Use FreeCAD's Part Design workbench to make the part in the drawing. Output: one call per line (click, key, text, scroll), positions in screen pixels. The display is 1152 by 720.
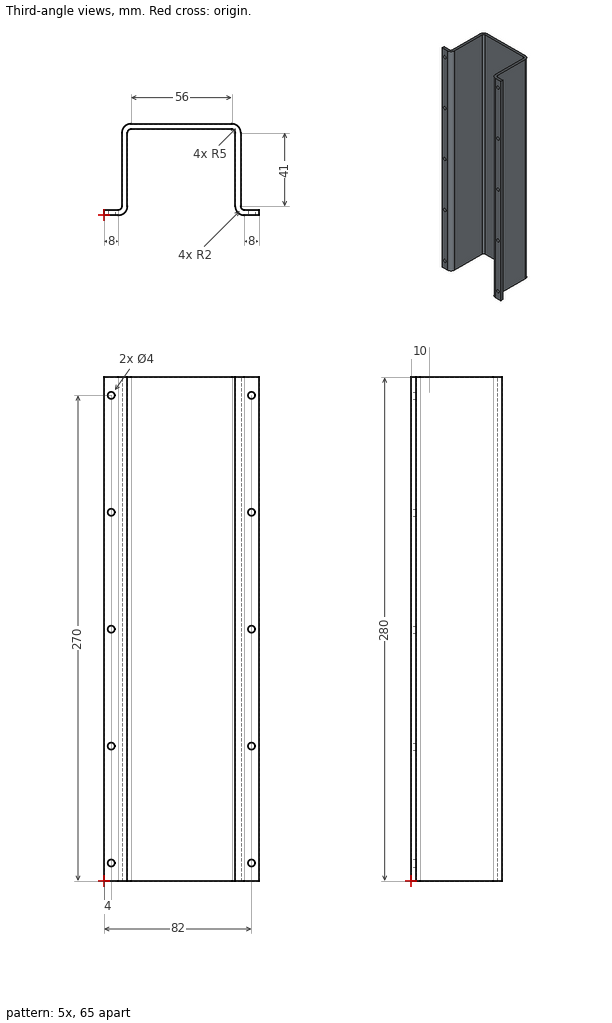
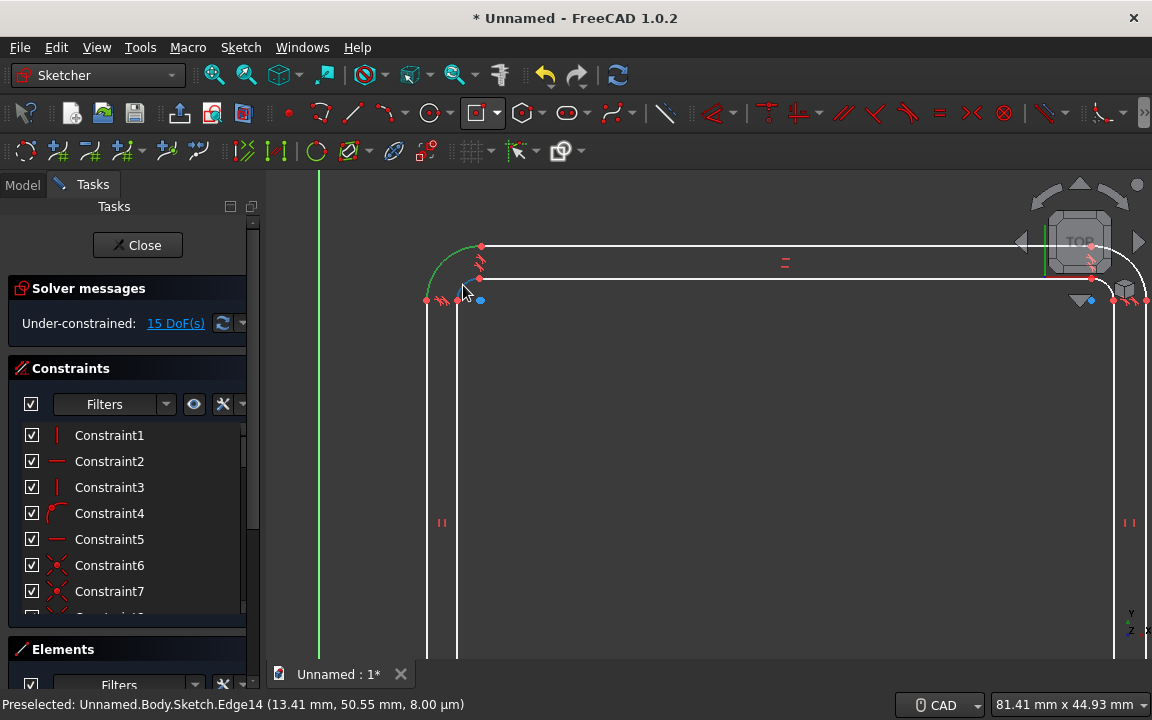
click(464, 285)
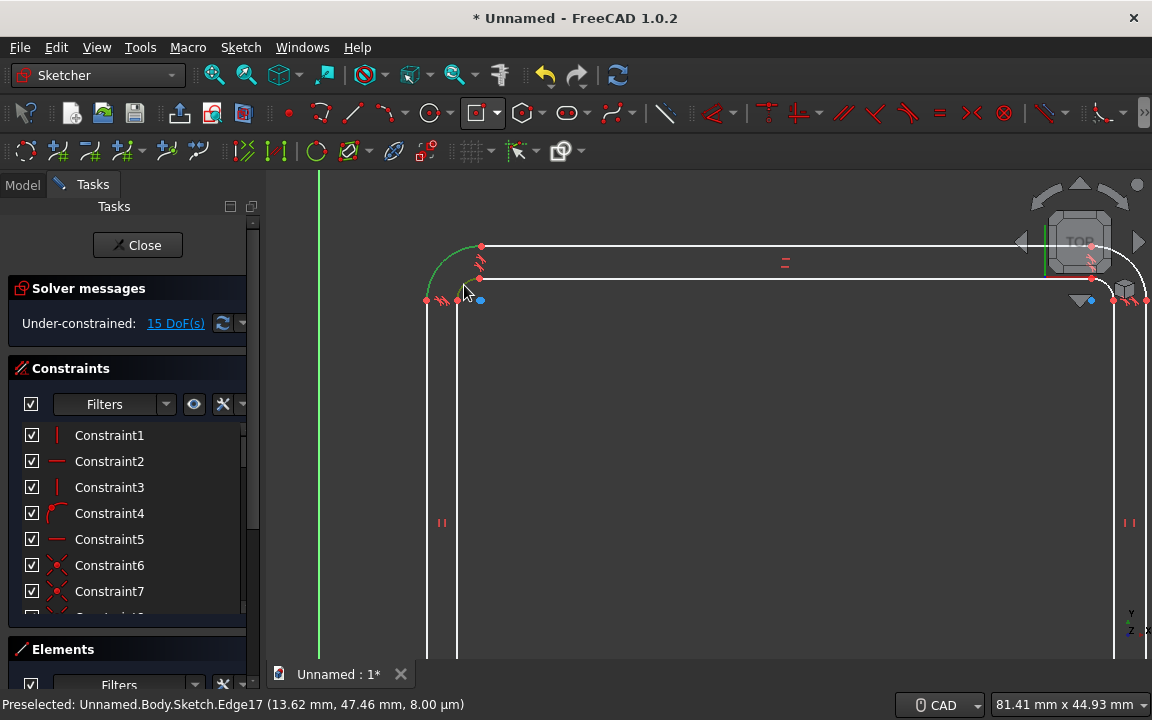
key(c)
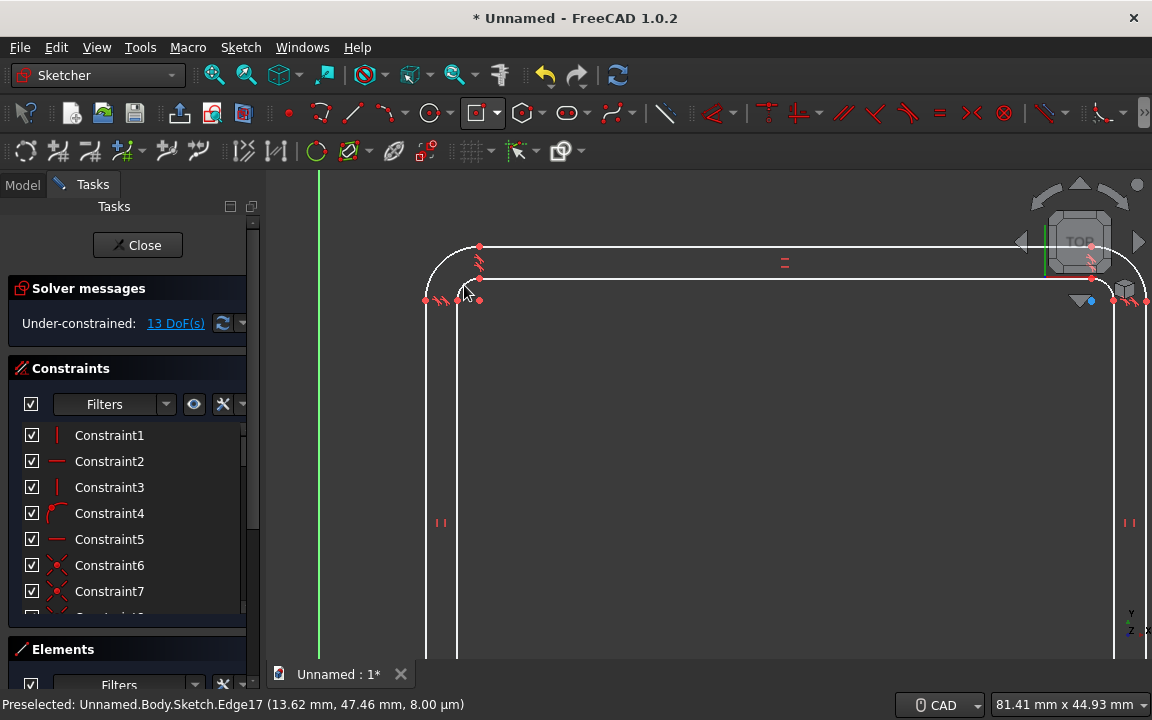
scroll(463, 285, down, 3)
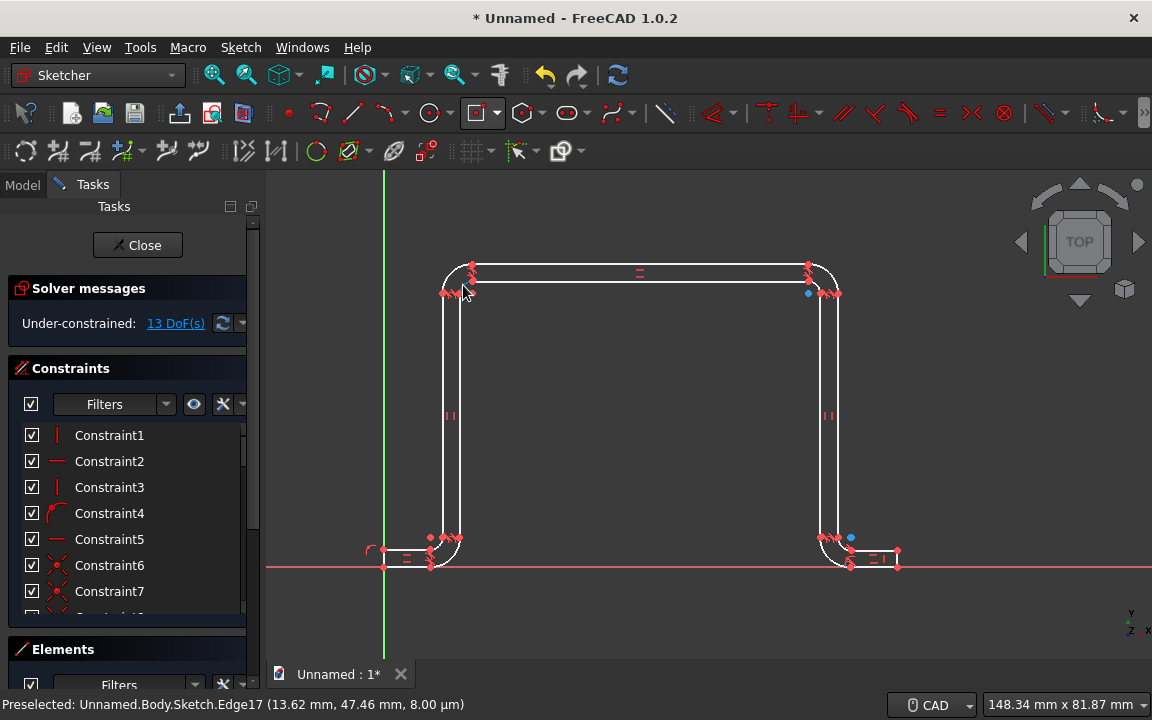
click(835, 280)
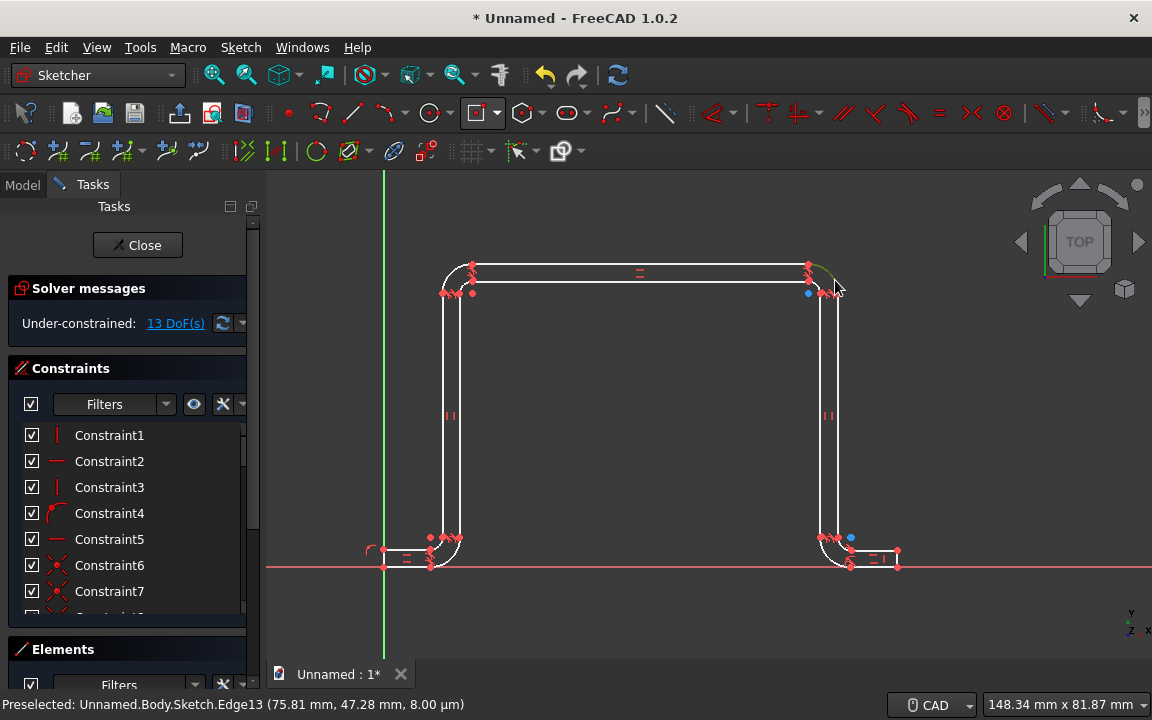
scroll(817, 285, up, 3)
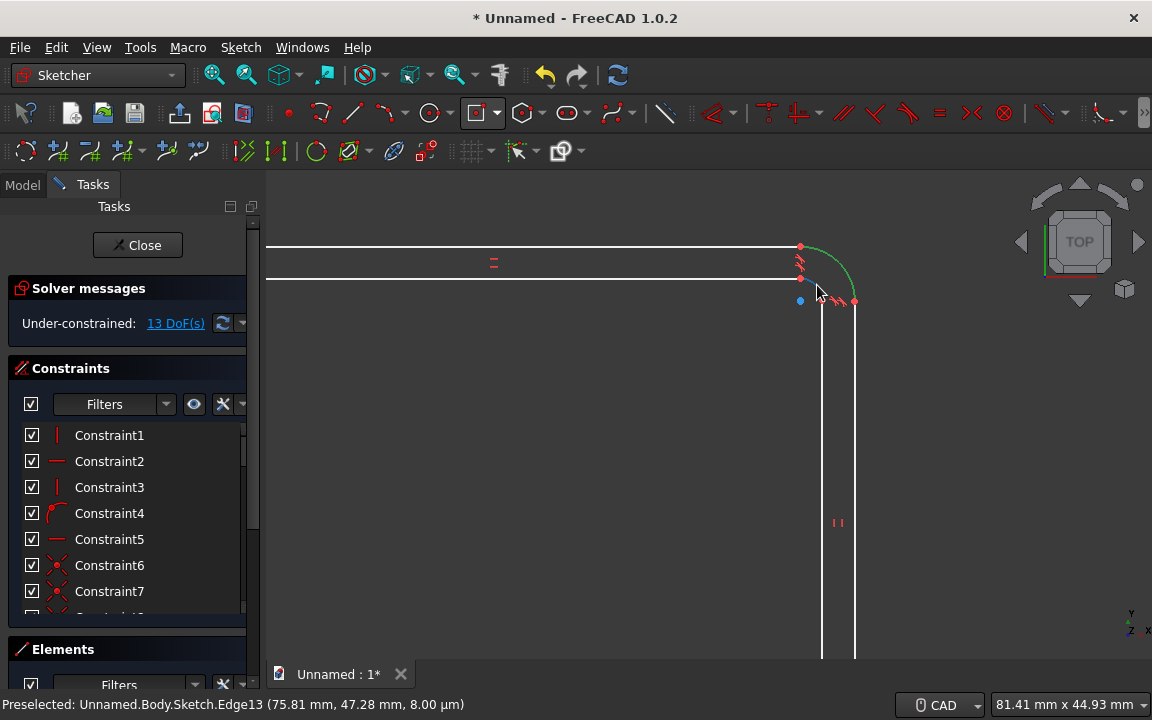
click(816, 285)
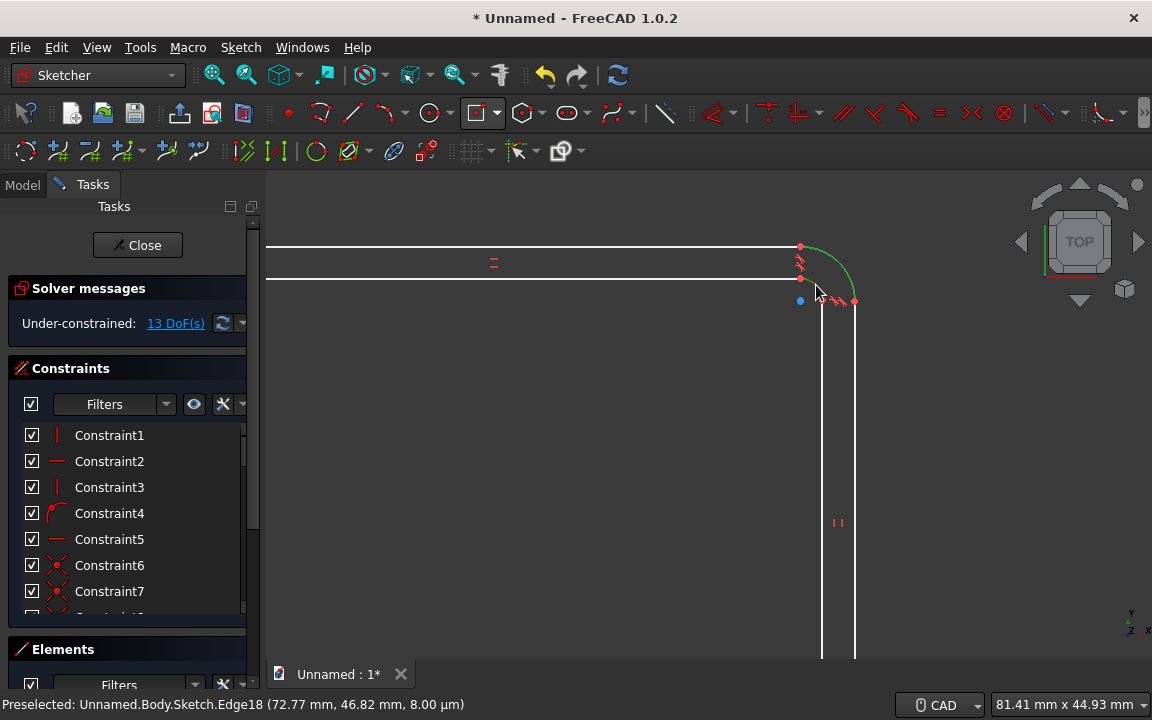
key(c)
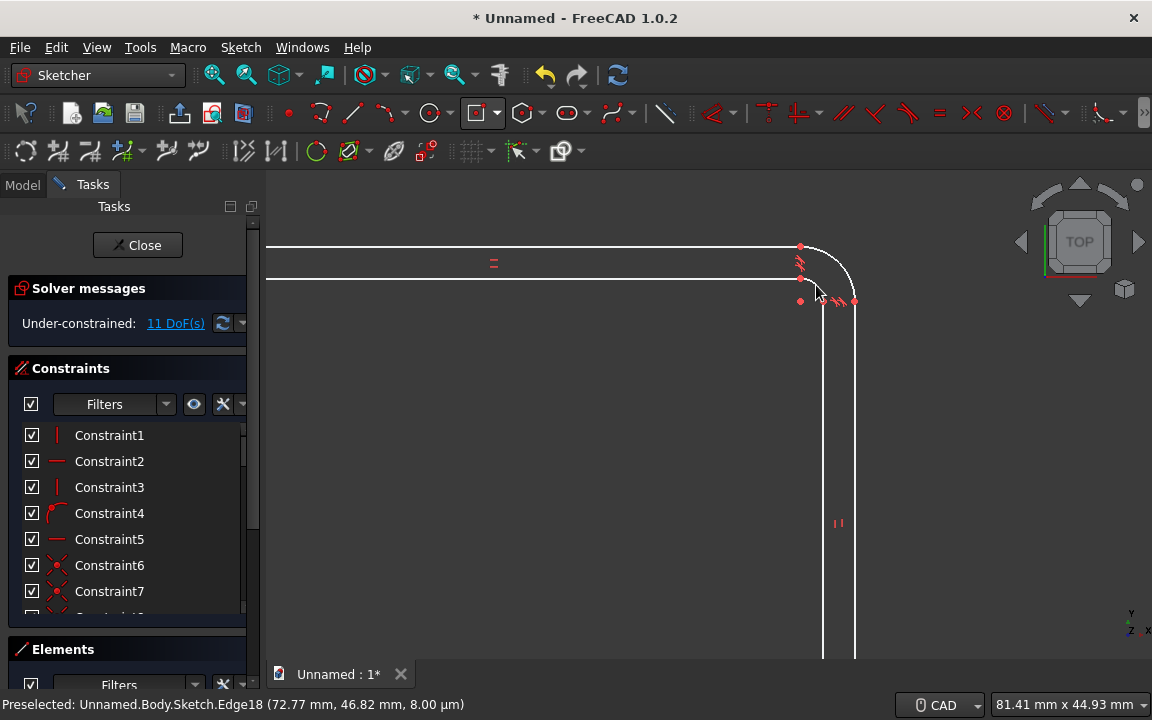
scroll(817, 285, down, 3)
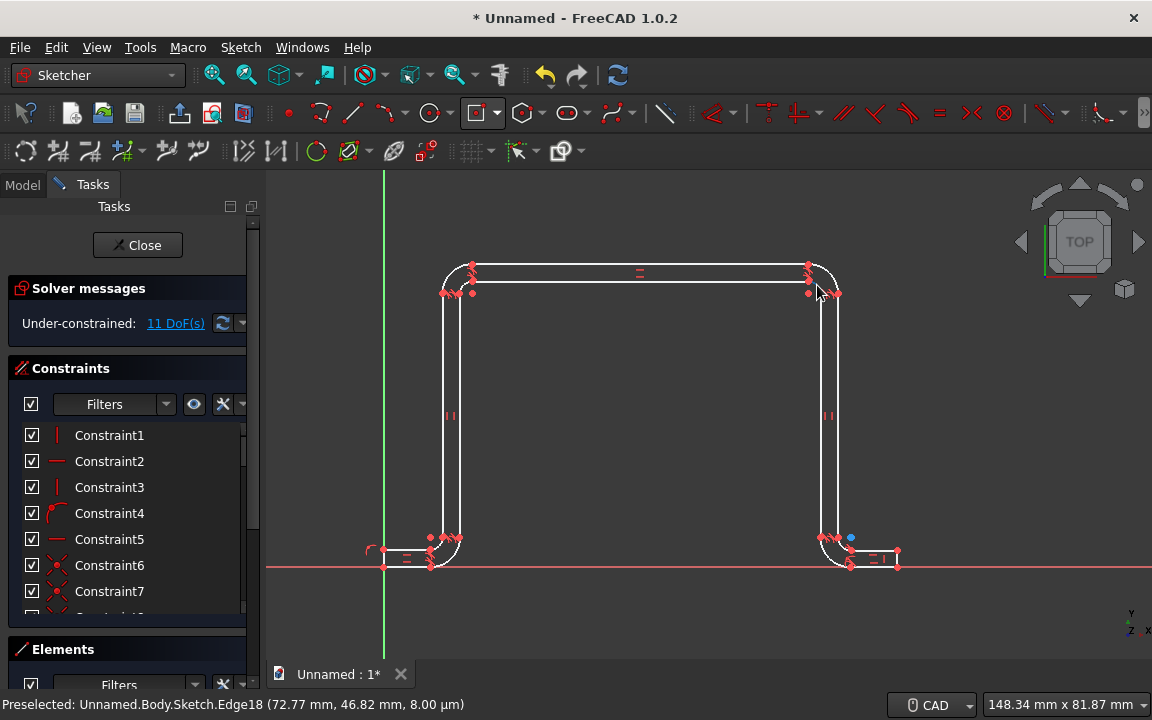
click(824, 551)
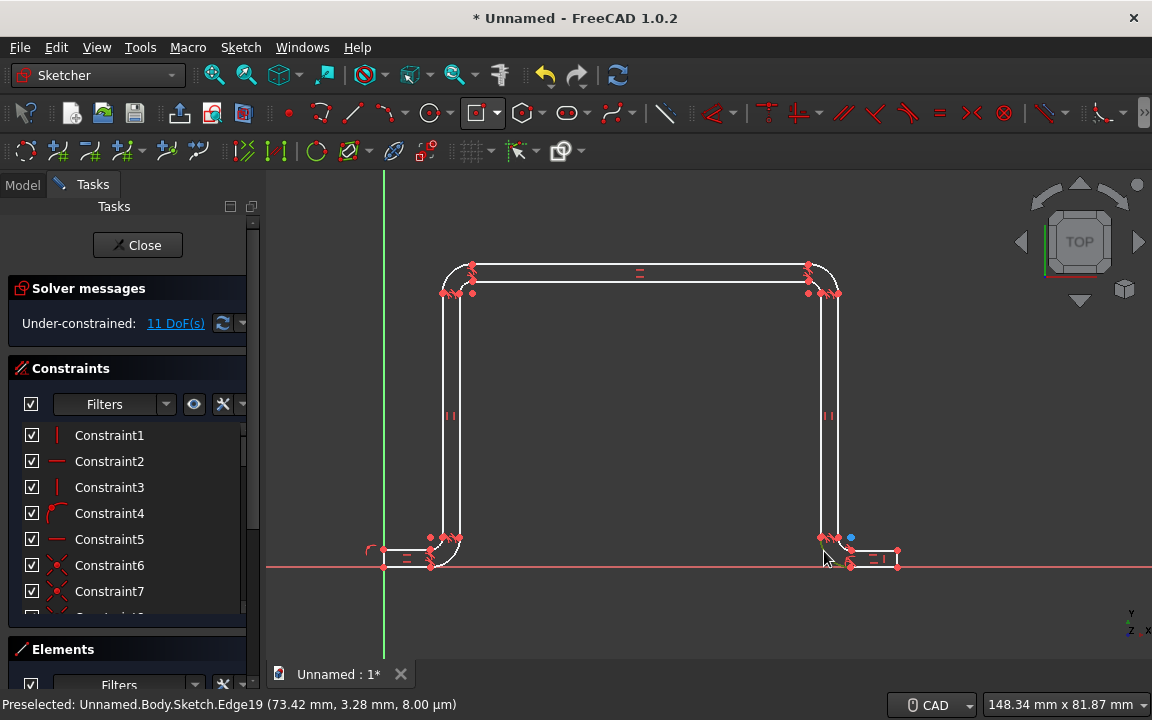
scroll(842, 547, up, 2)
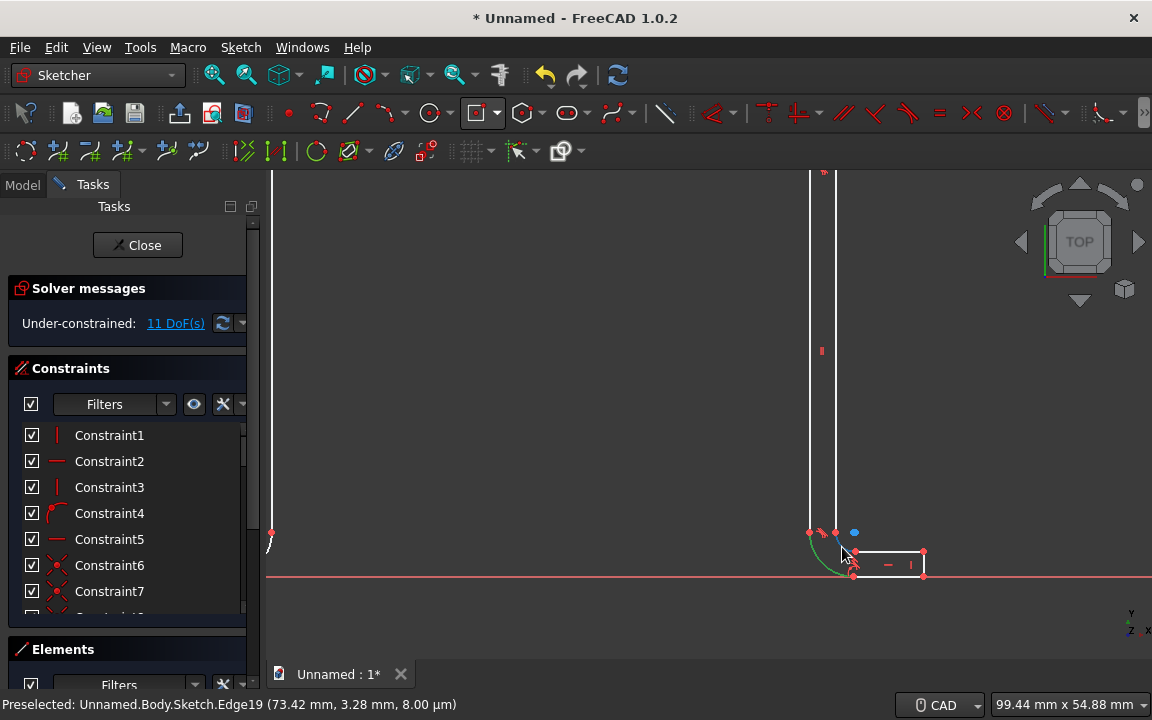
click(842, 546)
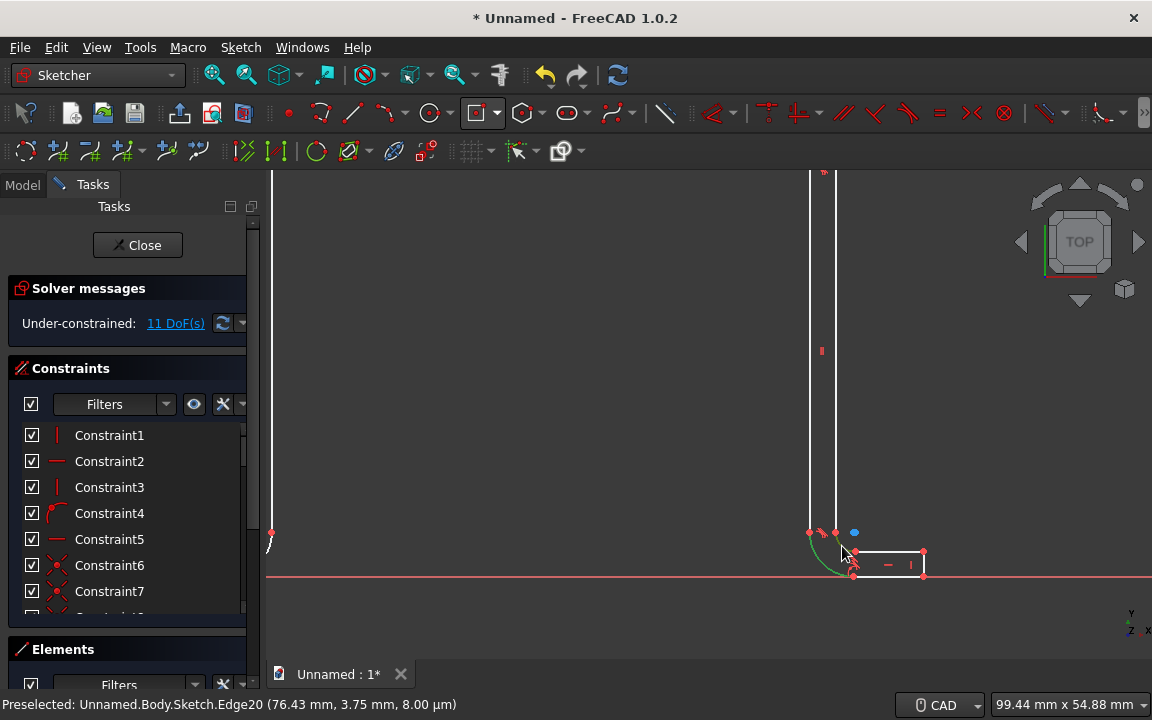
click(768, 114)